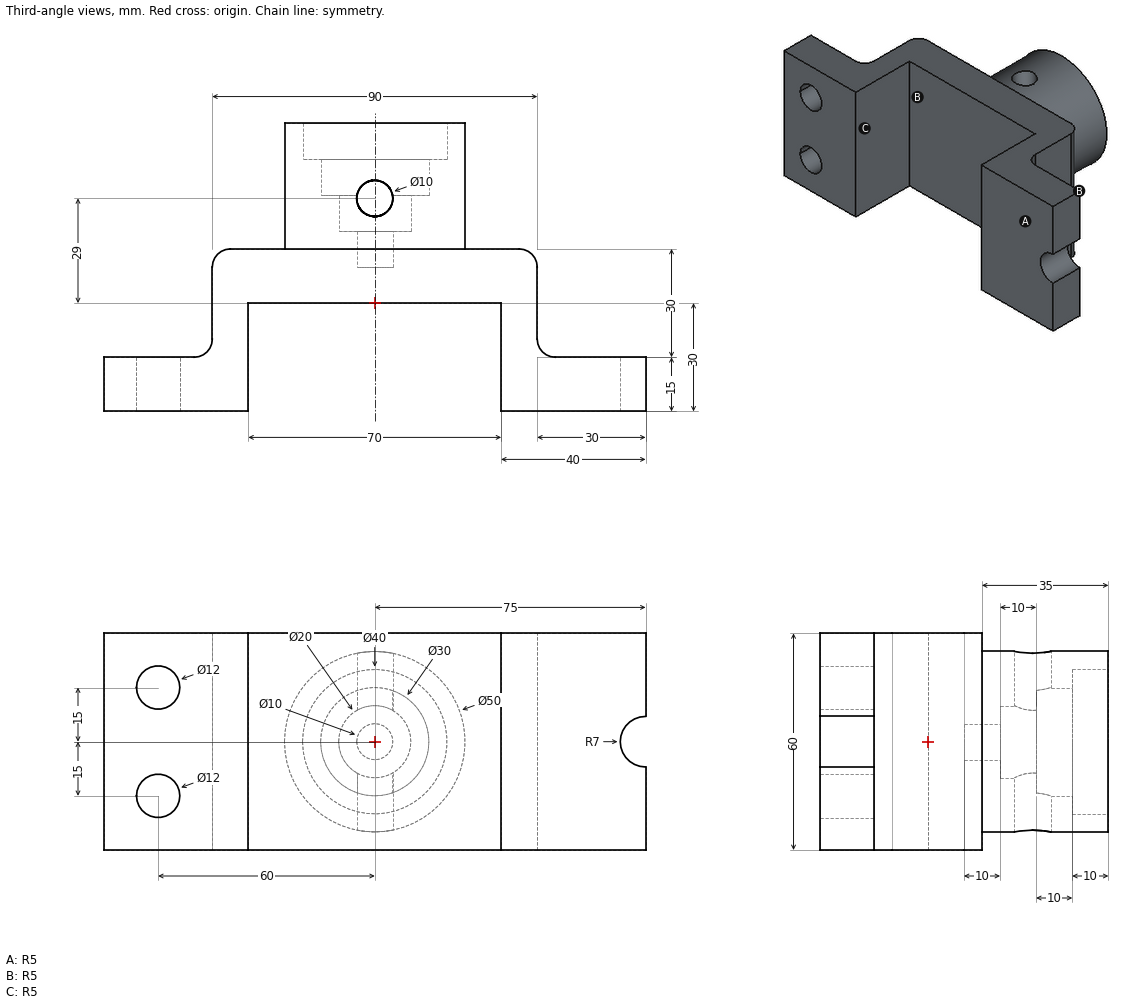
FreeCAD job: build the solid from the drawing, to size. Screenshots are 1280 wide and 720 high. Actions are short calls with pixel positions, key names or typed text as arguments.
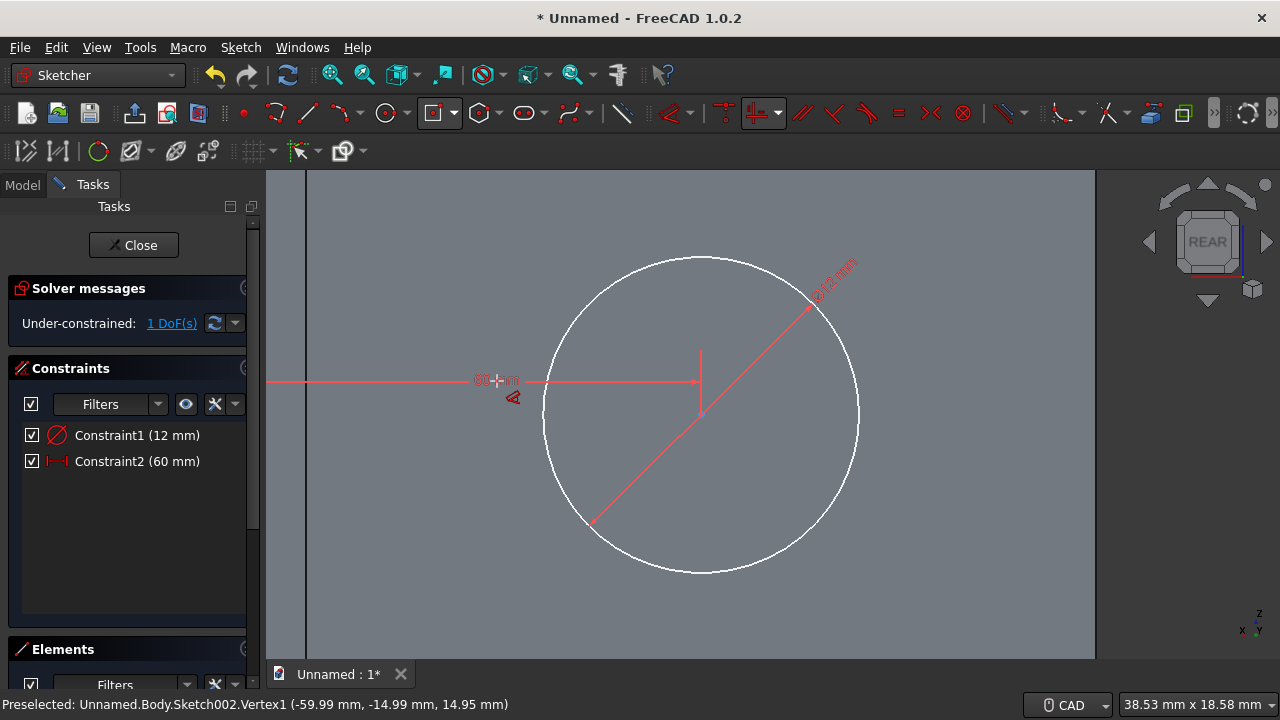
click(701, 415)
click(735, 523)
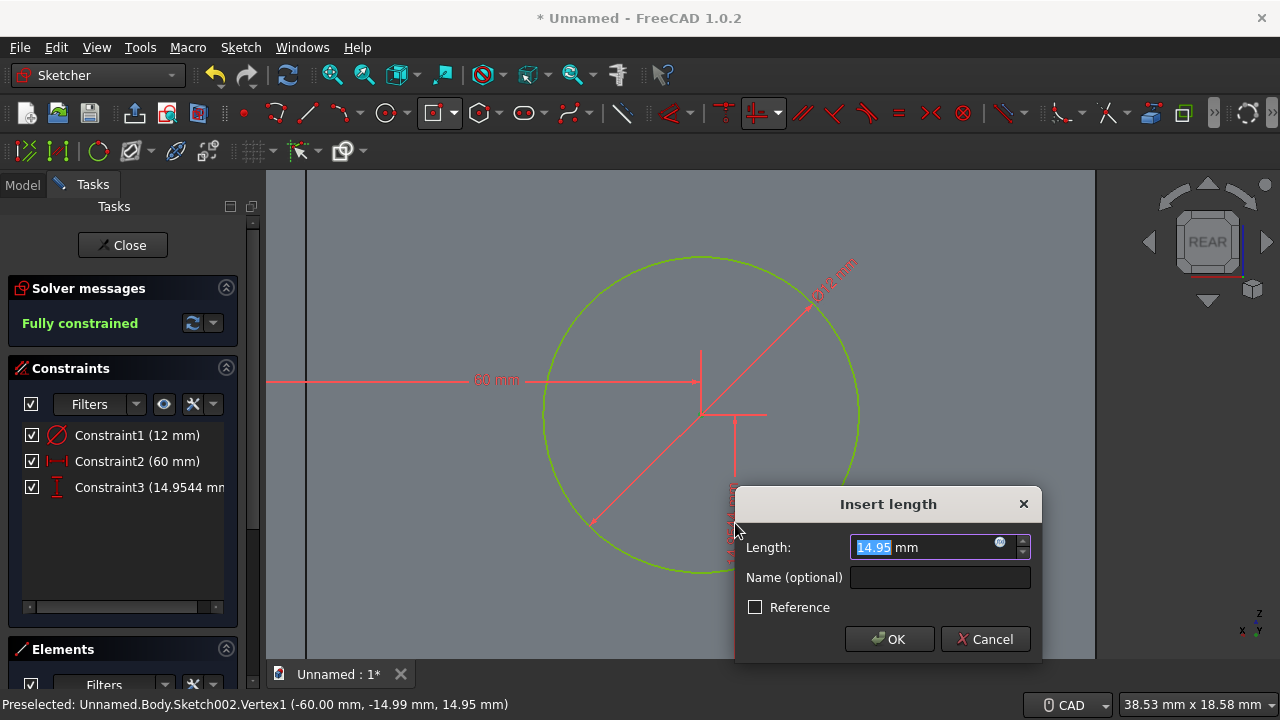
text(15)
key(Return)
key(Escape)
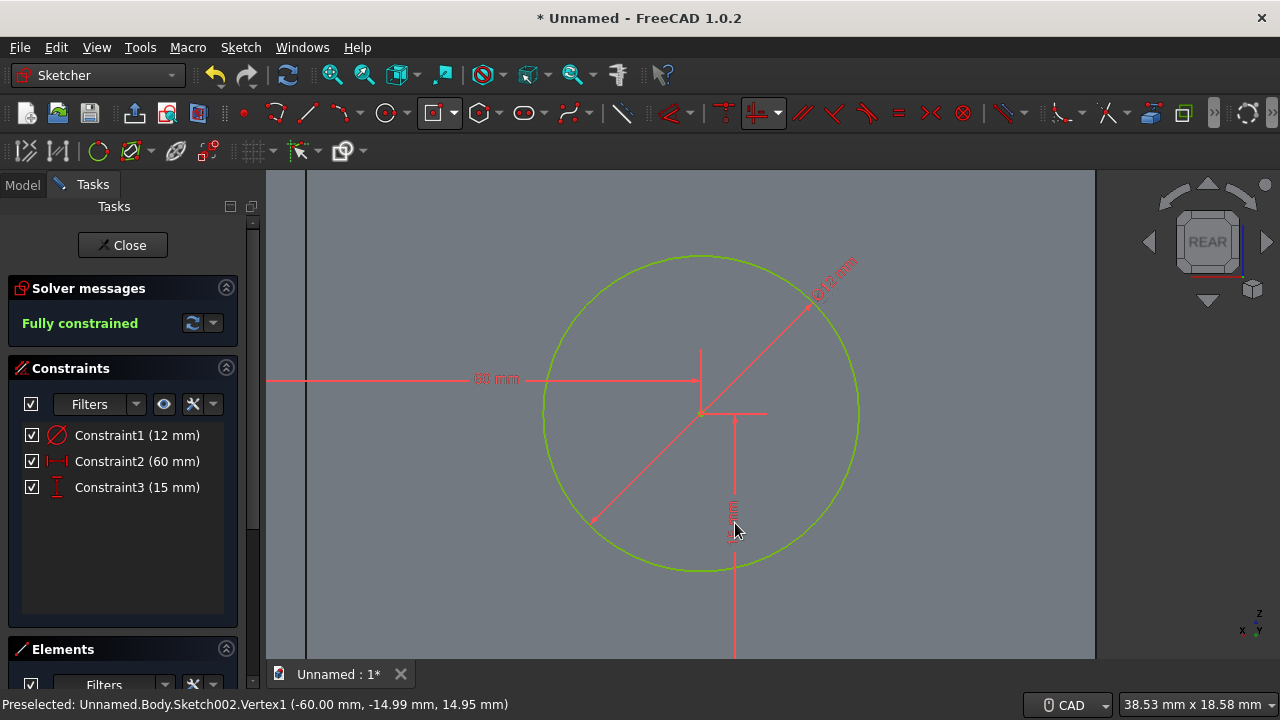
click(123, 245)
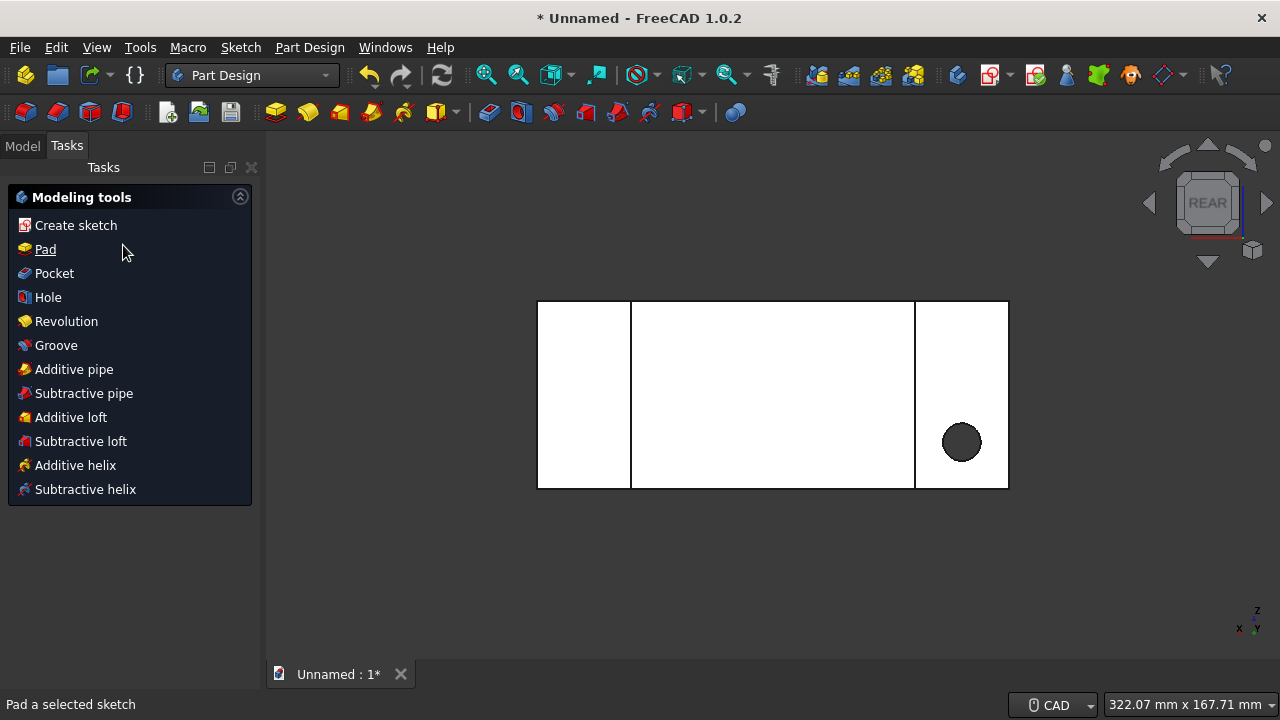
click(490, 112)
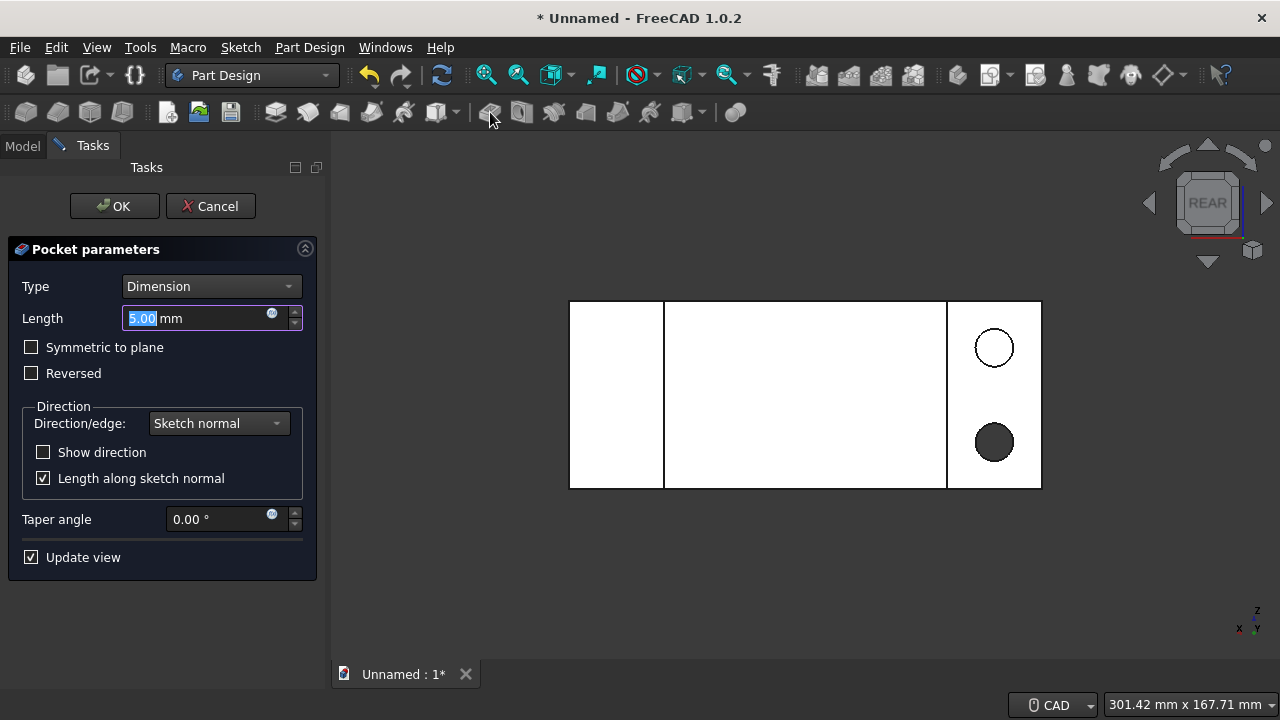
click(212, 286)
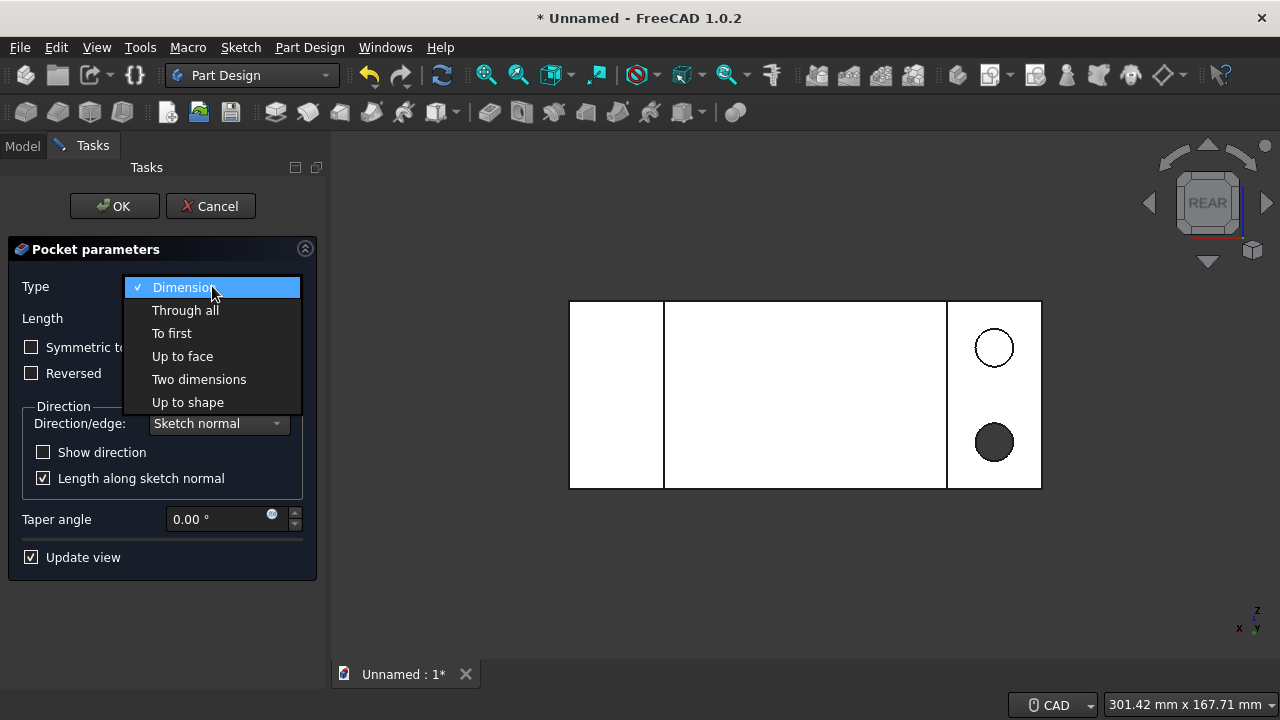
click(212, 334)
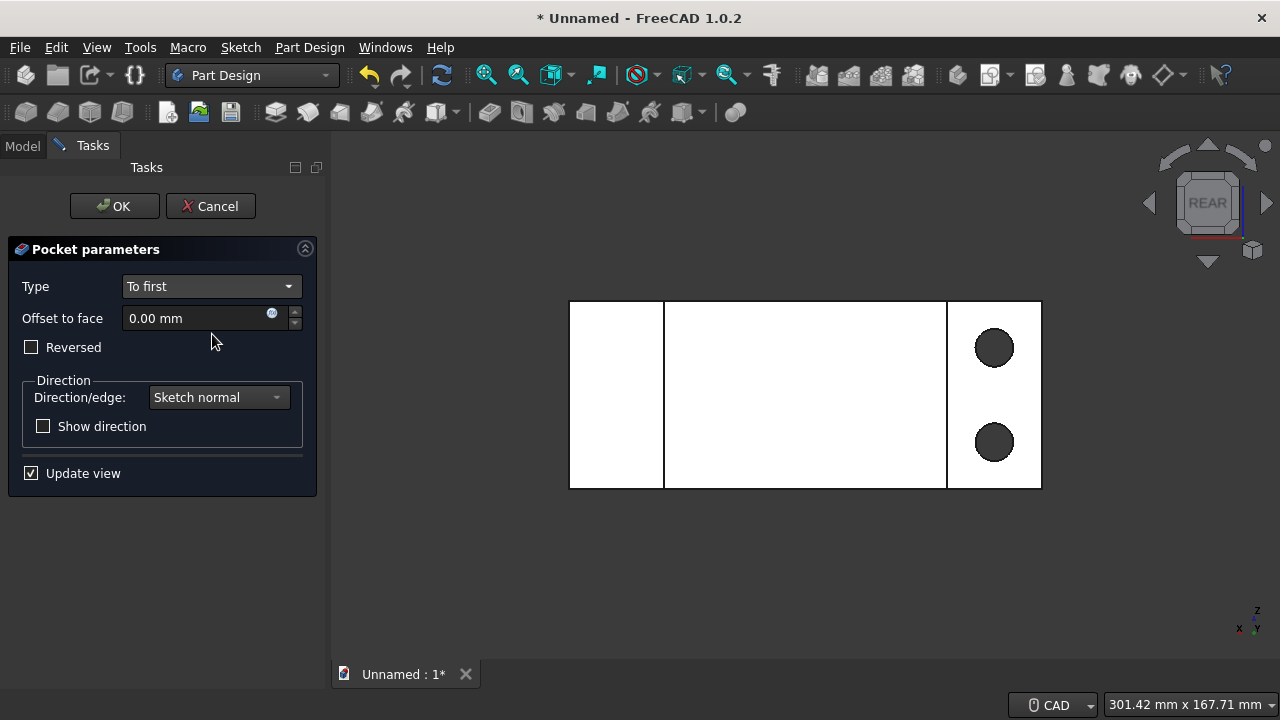
click(115, 206)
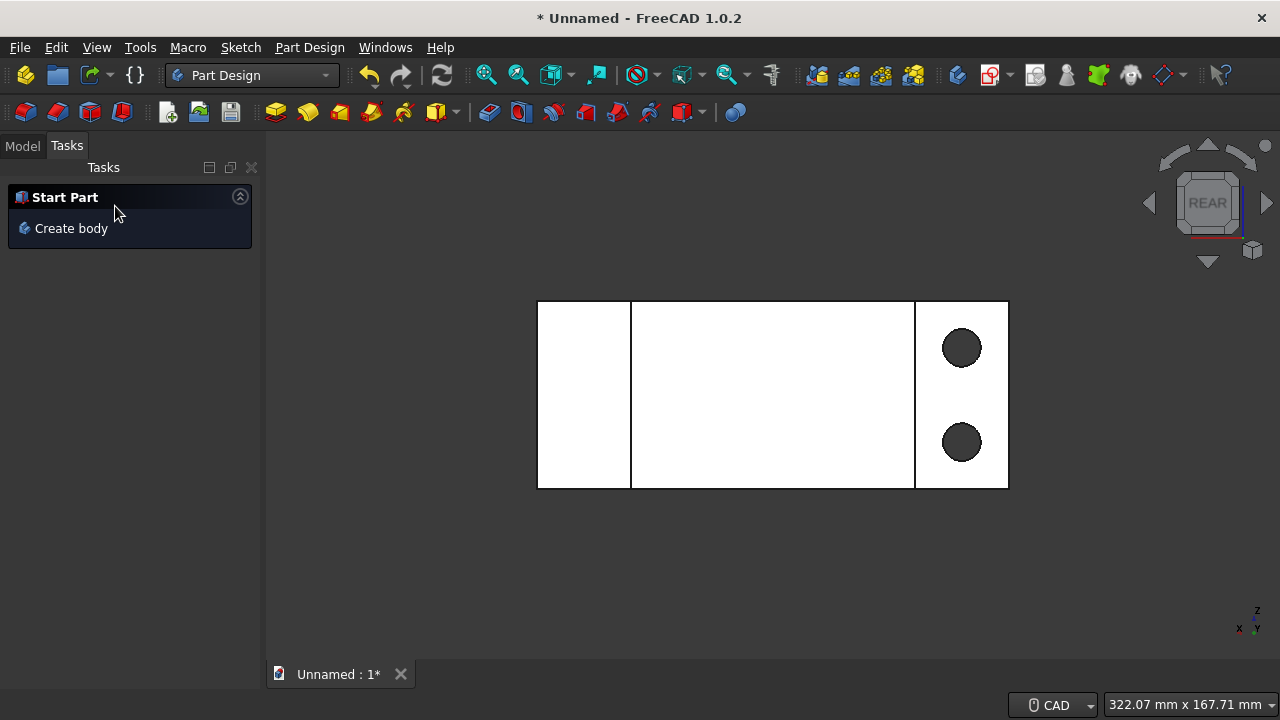
click(584, 367)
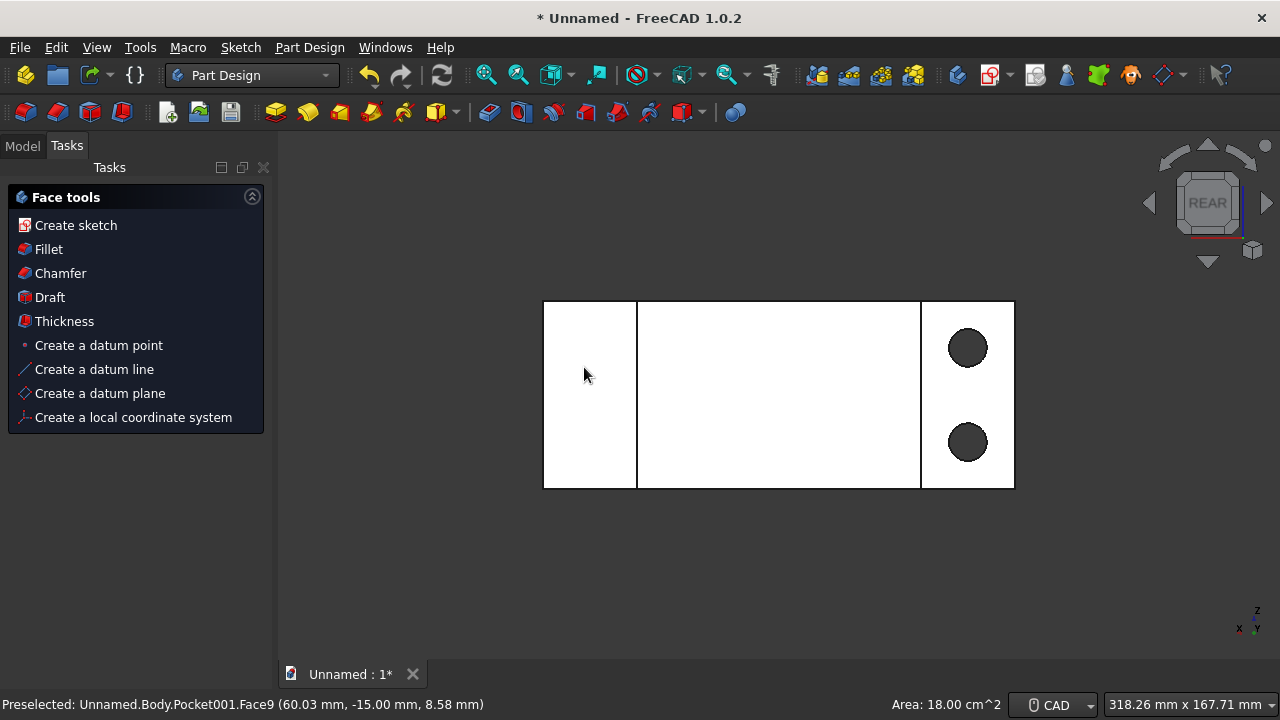
click(990, 76)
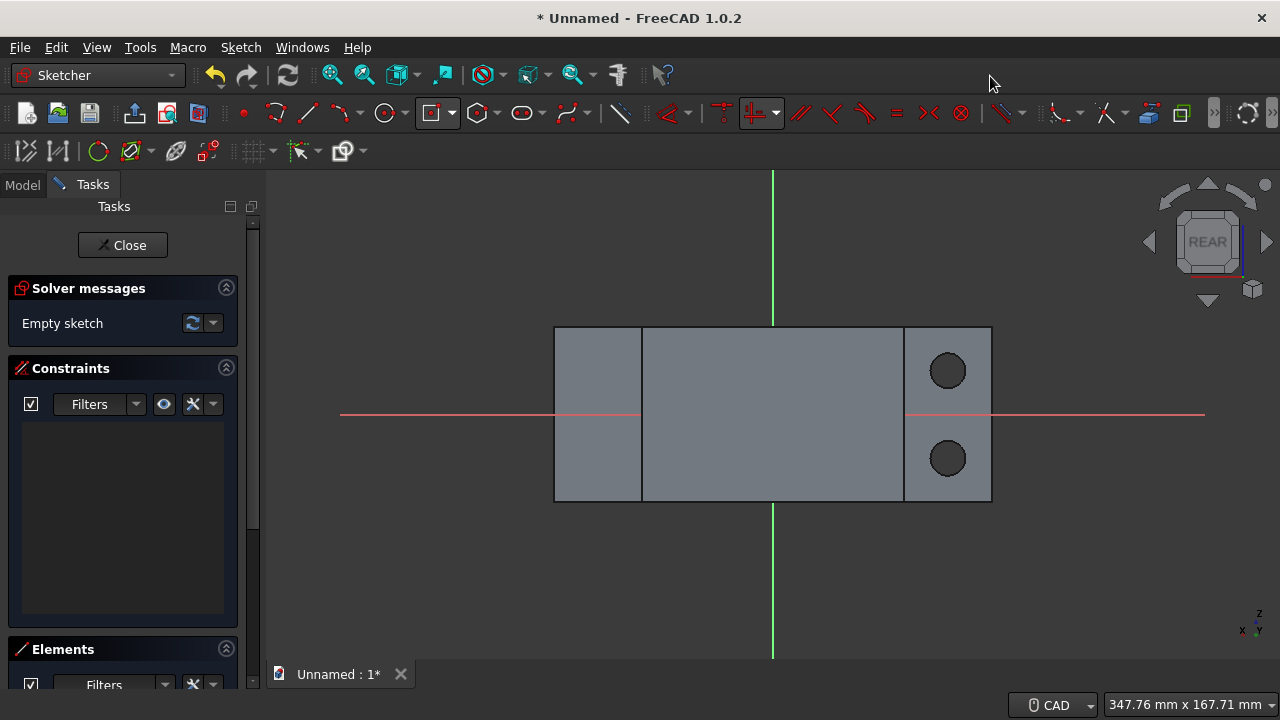
click(200, 114)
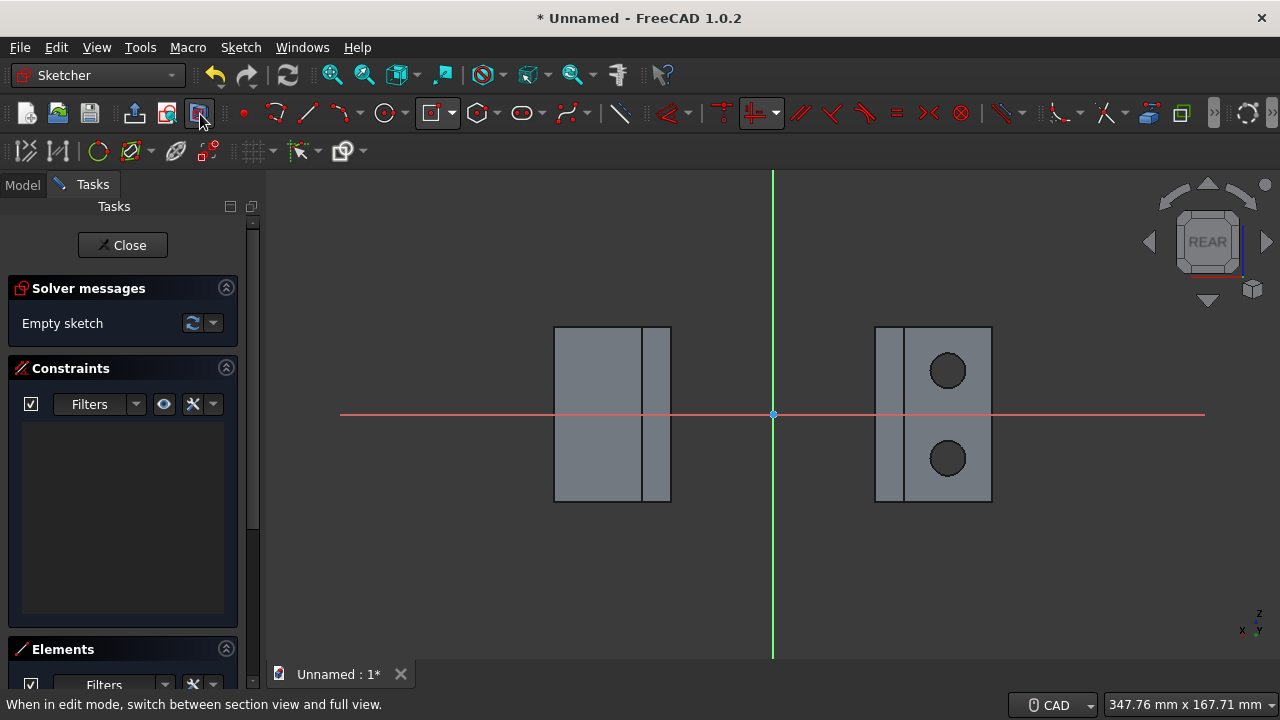
scroll(543, 415, up, 10)